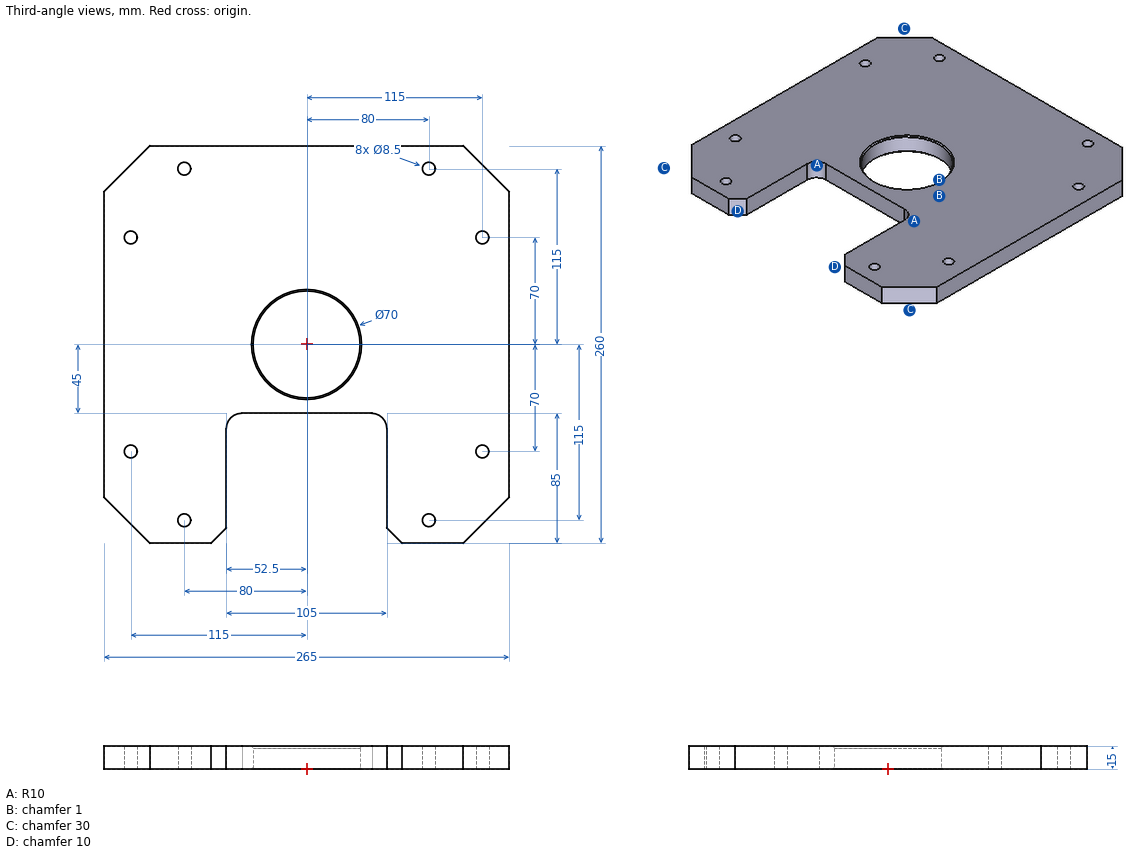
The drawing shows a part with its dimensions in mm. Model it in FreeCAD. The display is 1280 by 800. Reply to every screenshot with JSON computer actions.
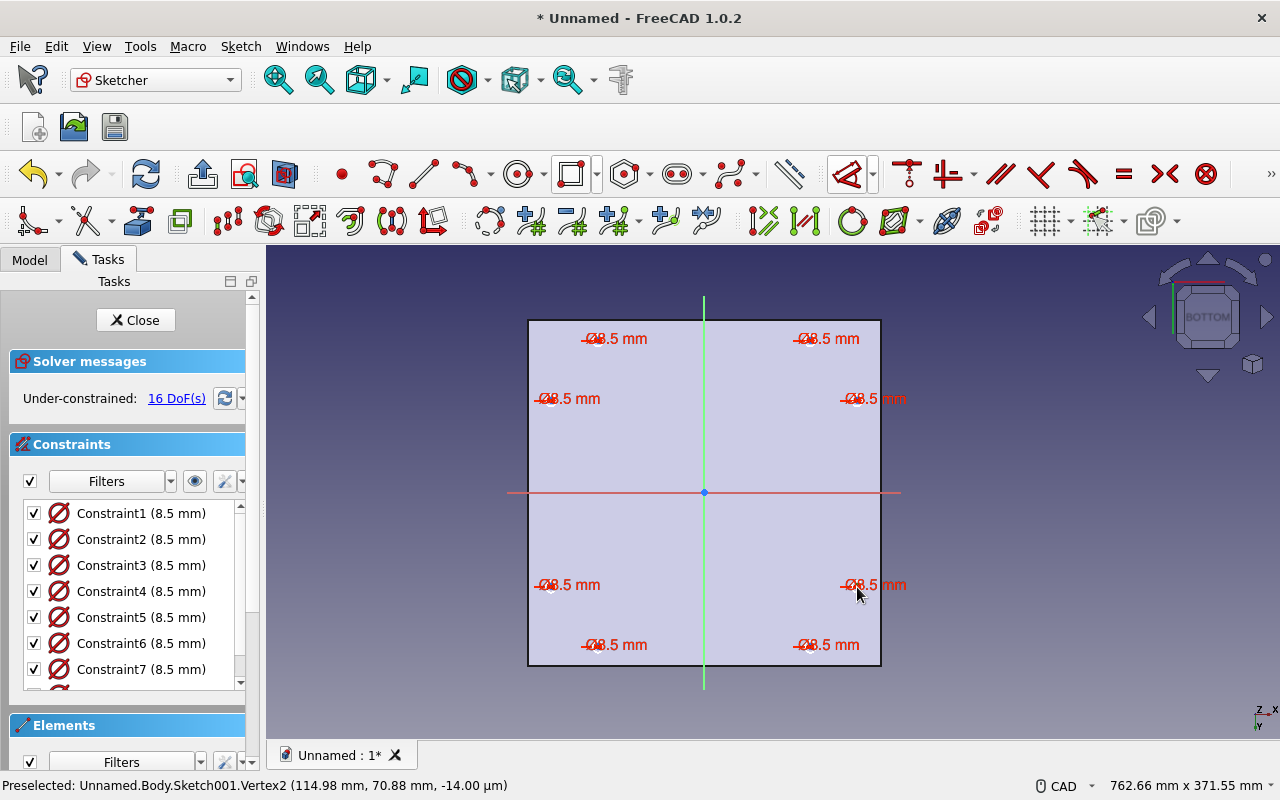
{"action": "left_click", "coordinate": [857, 401]}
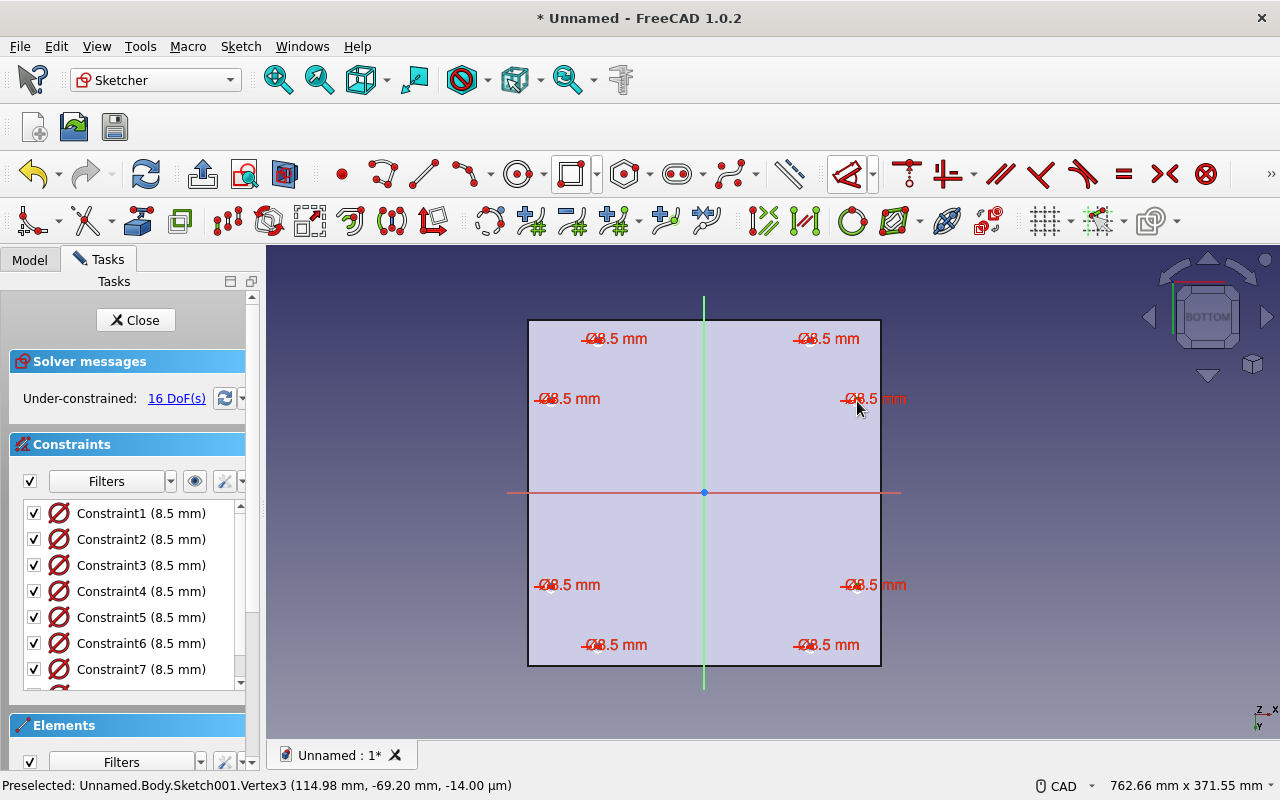
{"action": "left_click", "coordinate": [974, 174]}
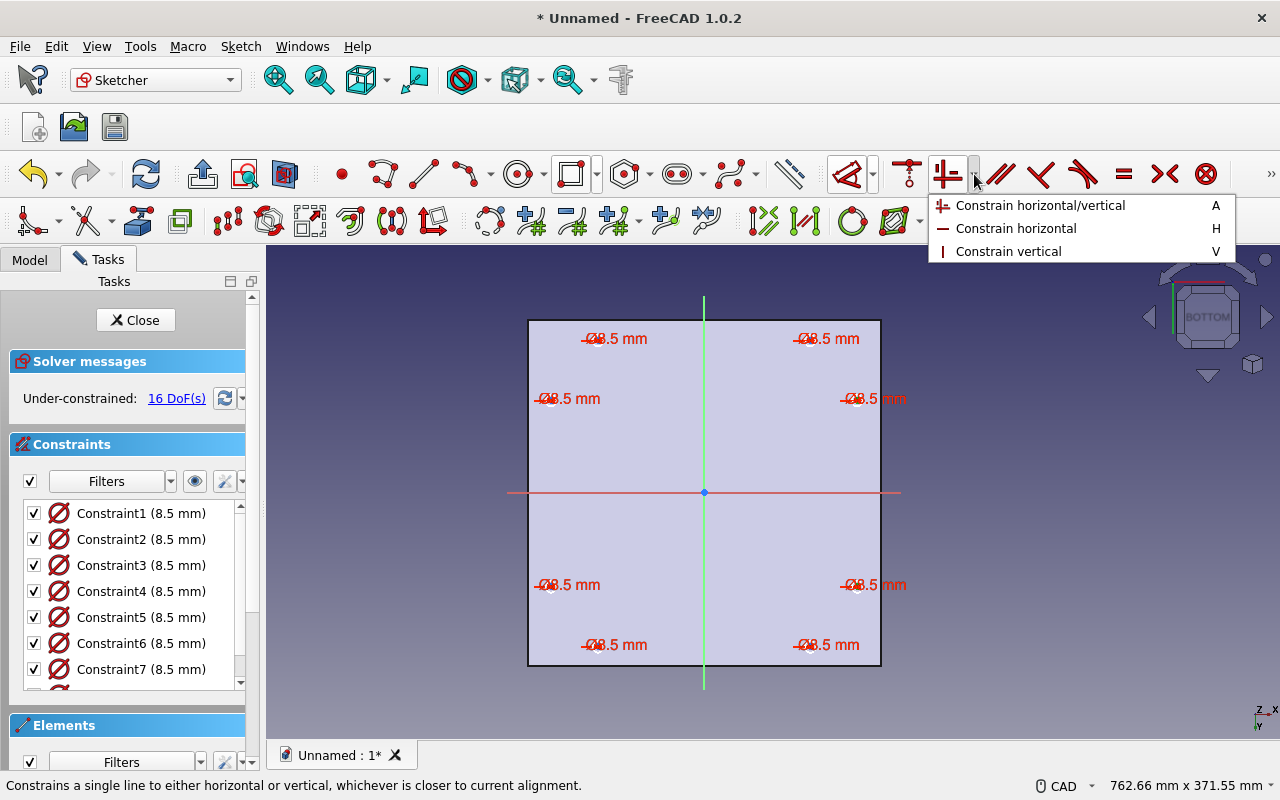
{"action": "left_click", "coordinate": [1082, 252]}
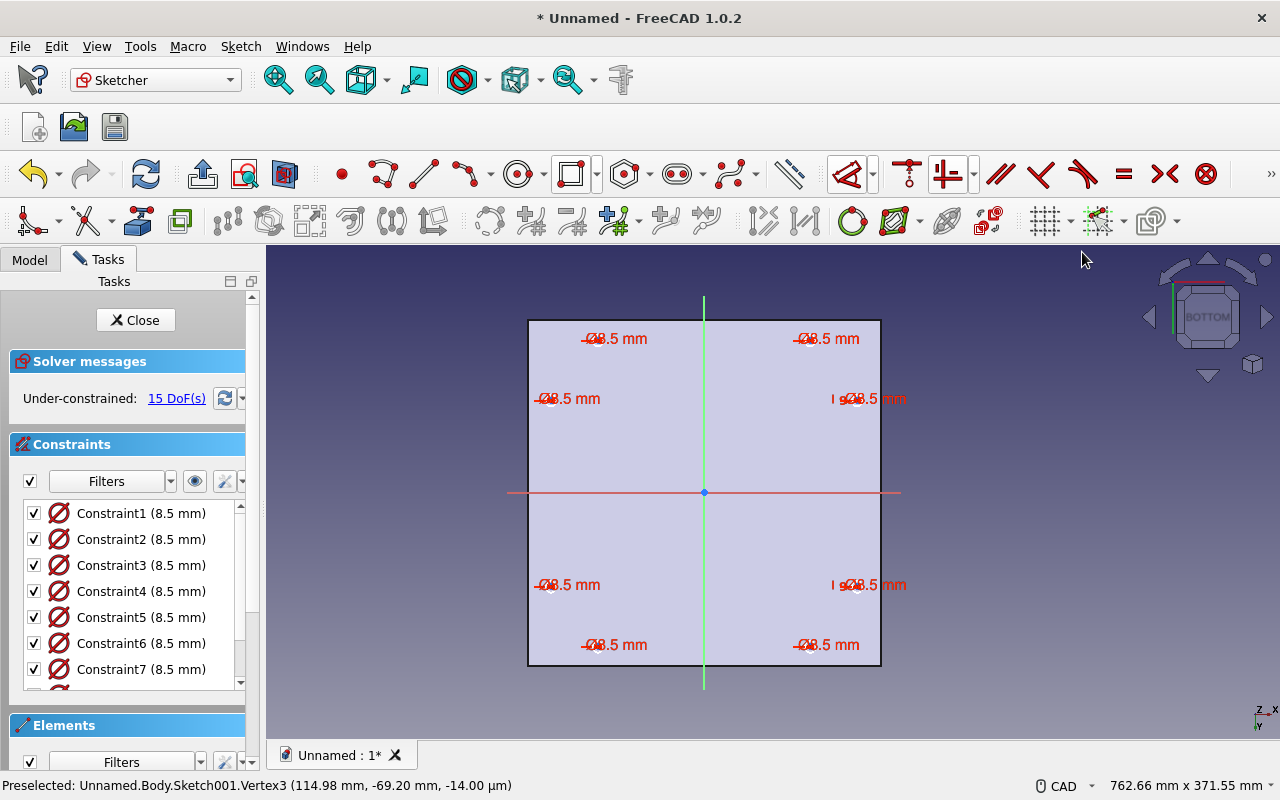
{"action": "left_click", "coordinate": [810, 647]}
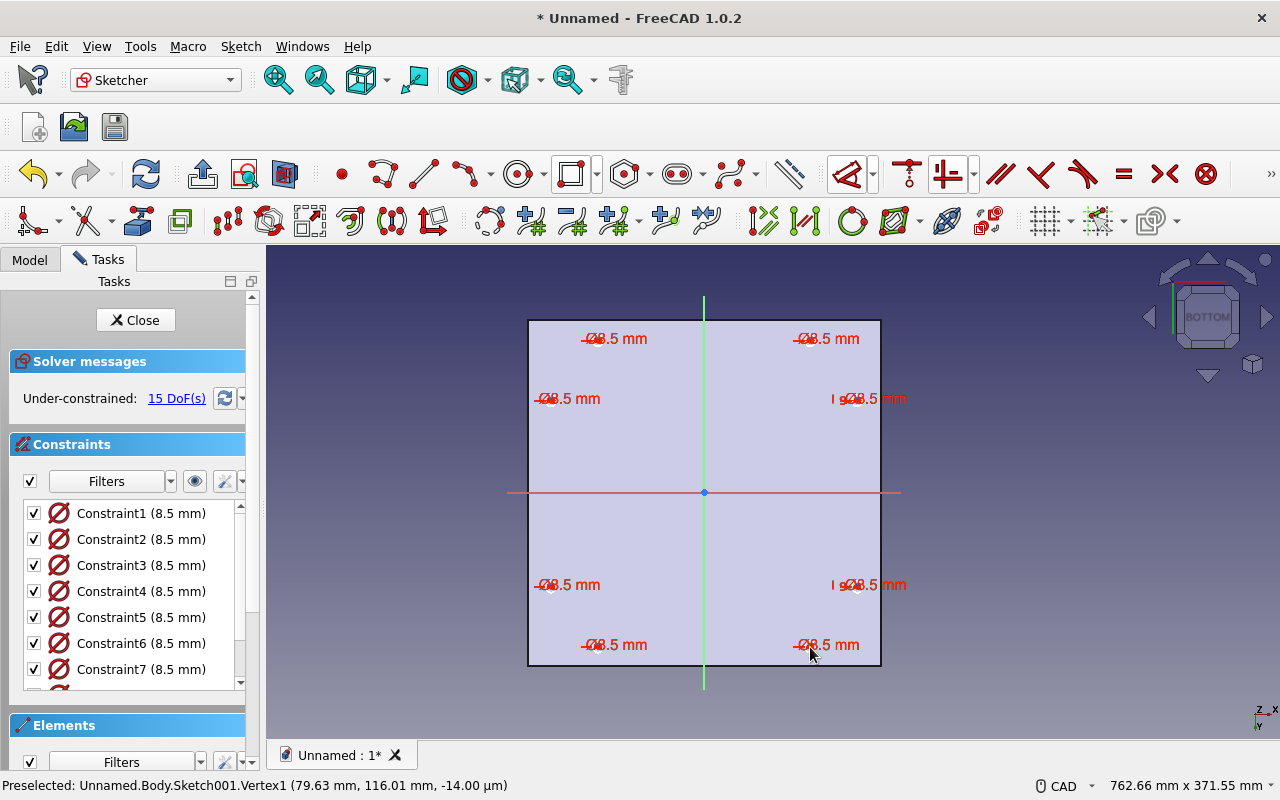
{"action": "left_click", "coordinate": [810, 341]}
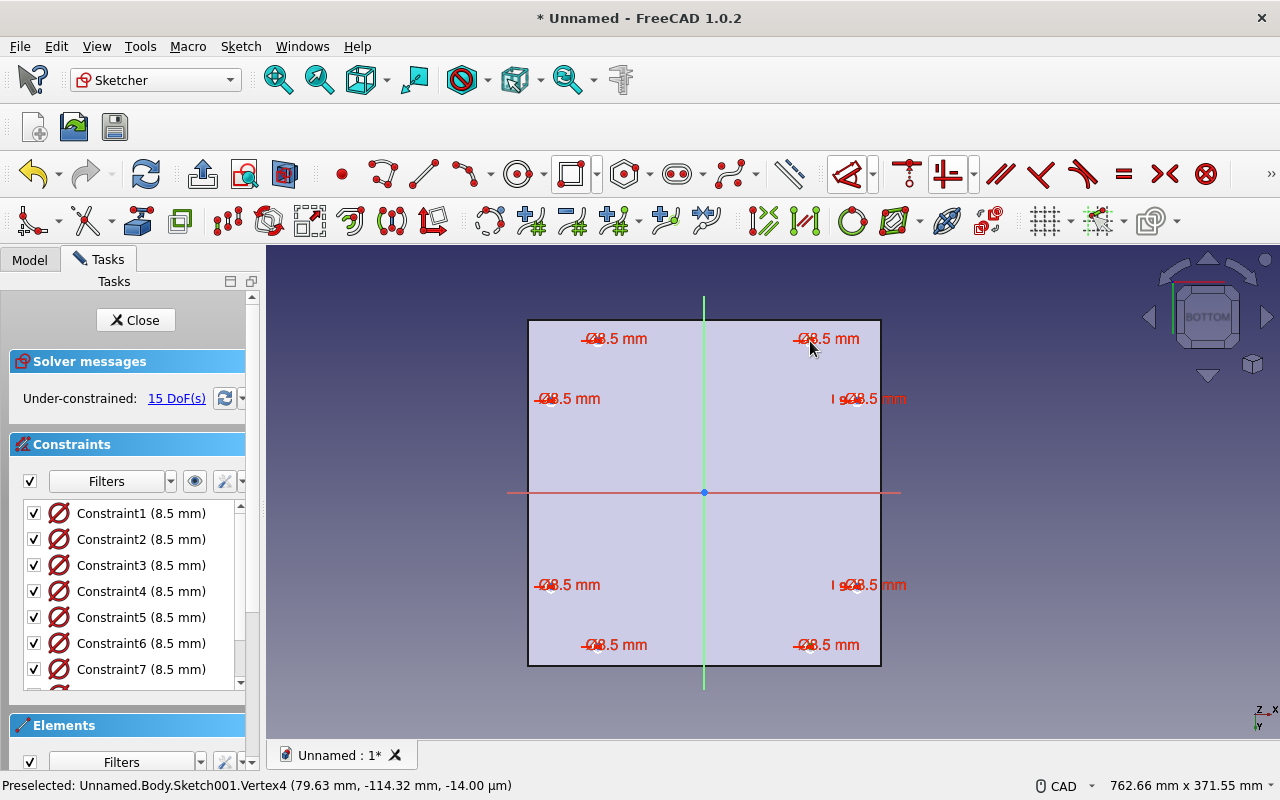
{"action": "left_click", "coordinate": [974, 174]}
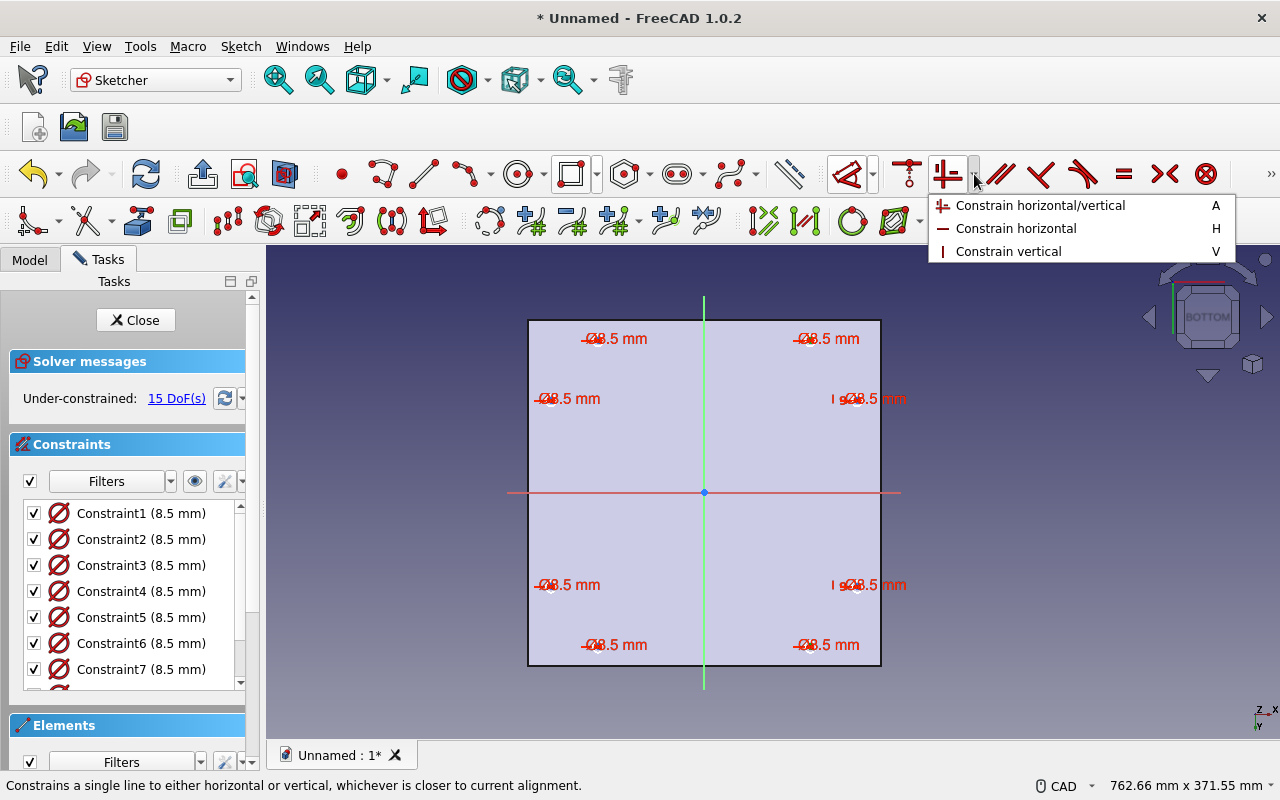
{"action": "left_click", "coordinate": [1082, 252]}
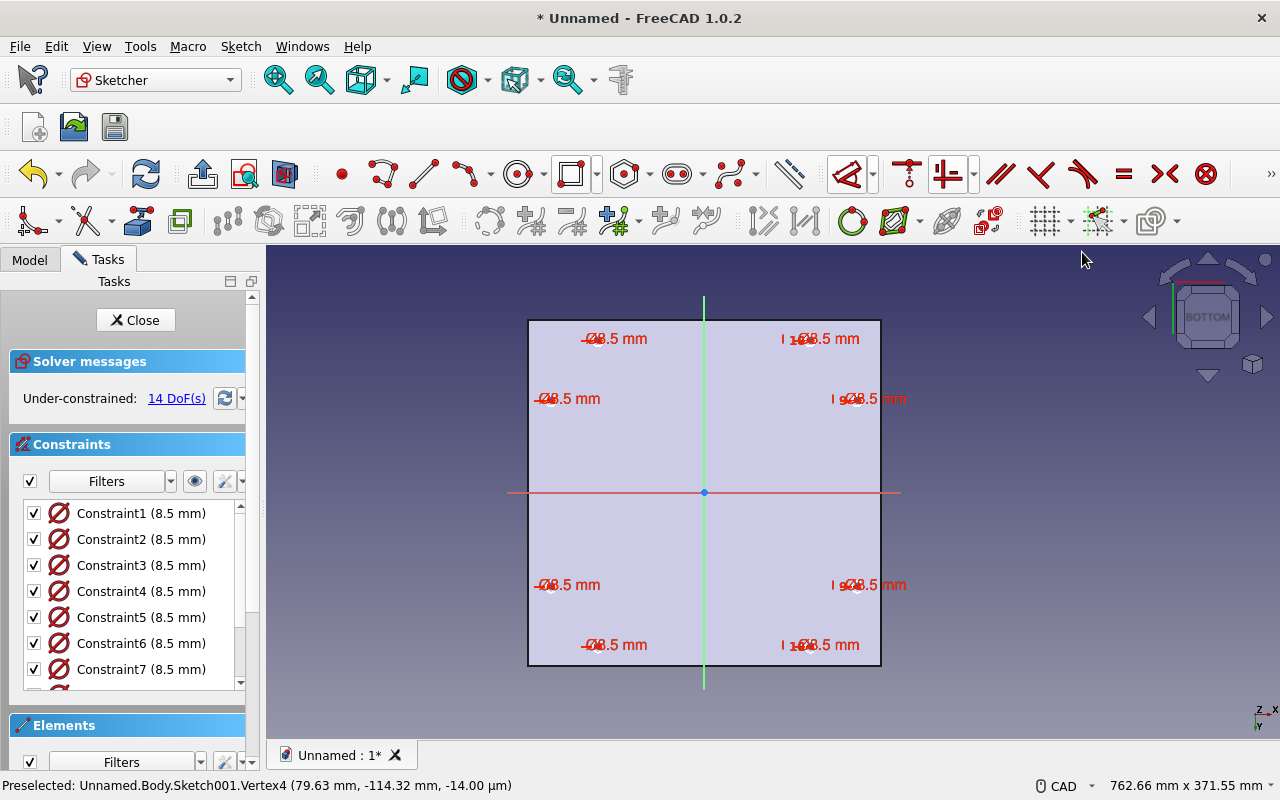
{"action": "left_click", "coordinate": [810, 341]}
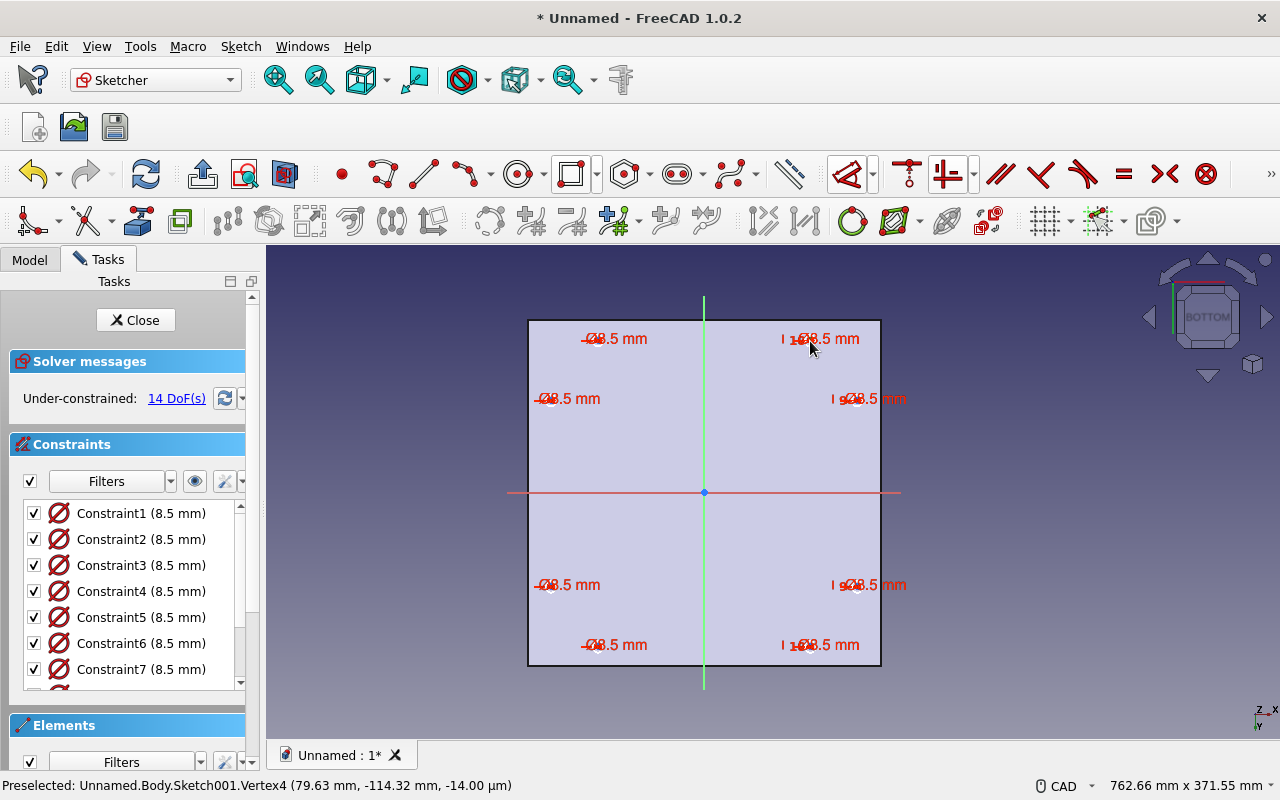
{"action": "left_click", "coordinate": [598, 341]}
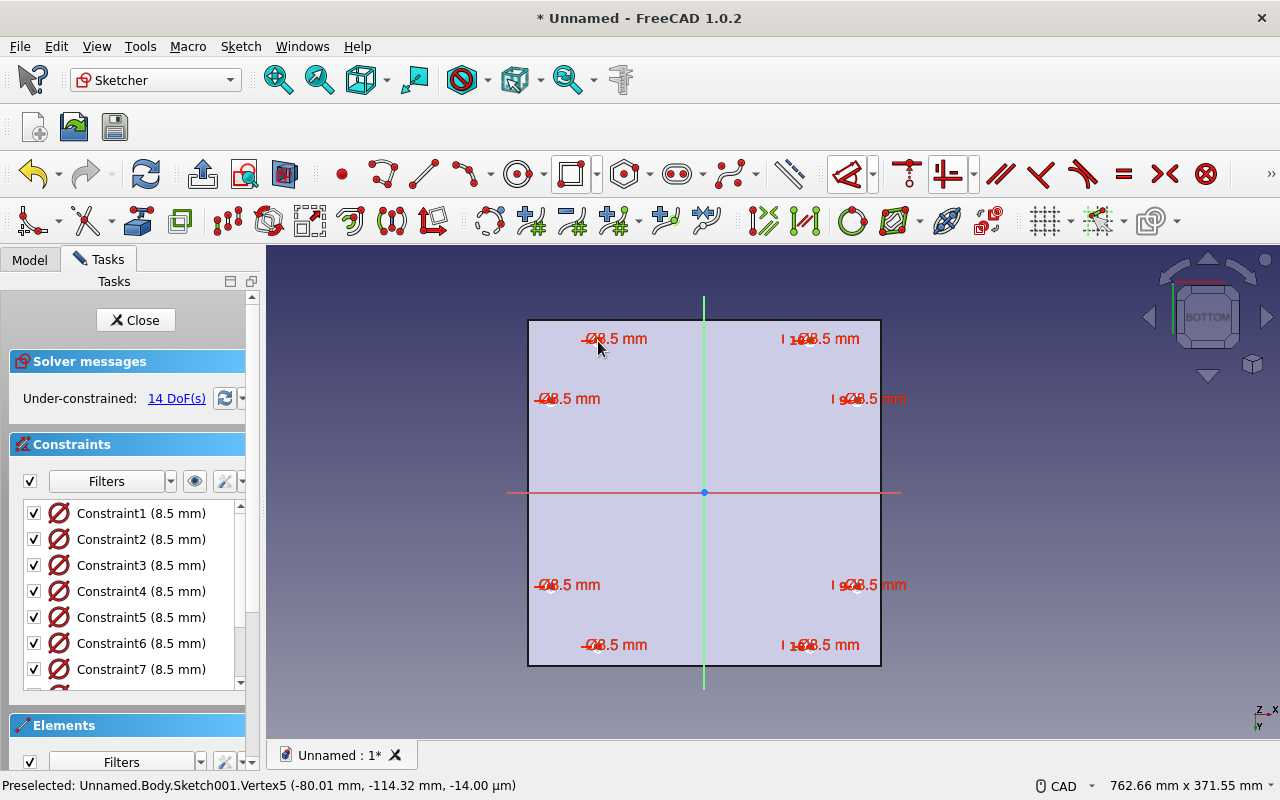
{"action": "key", "text": "h"}